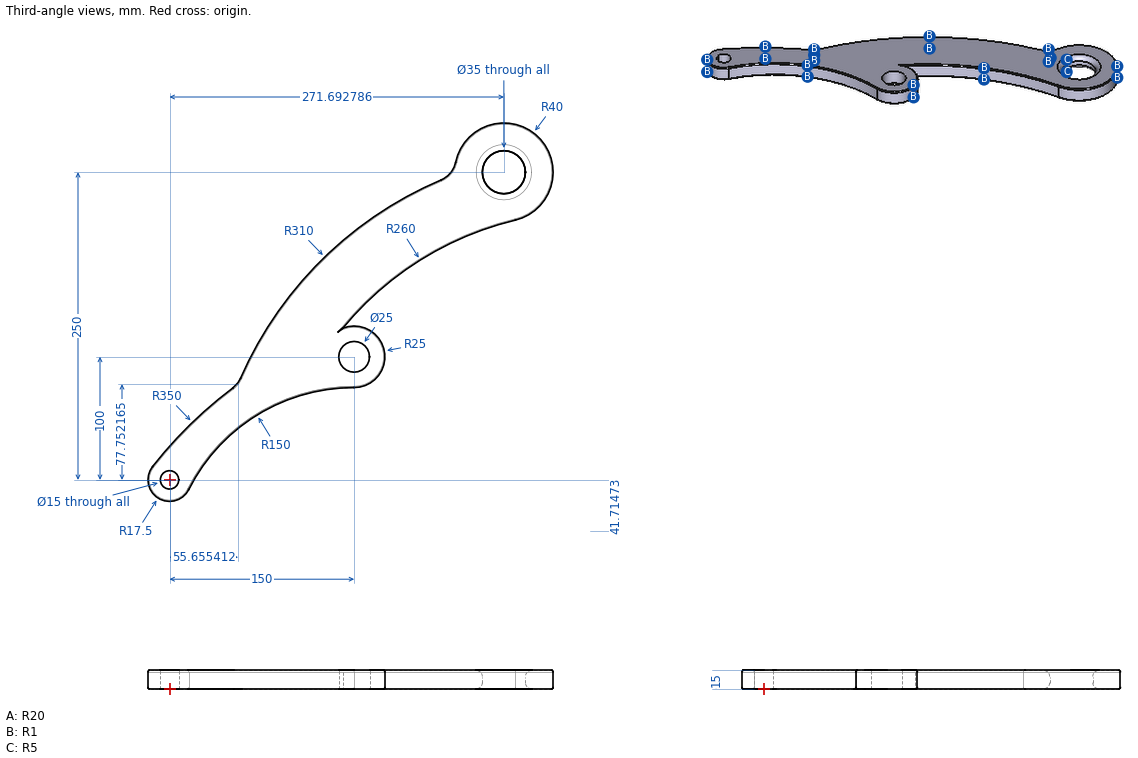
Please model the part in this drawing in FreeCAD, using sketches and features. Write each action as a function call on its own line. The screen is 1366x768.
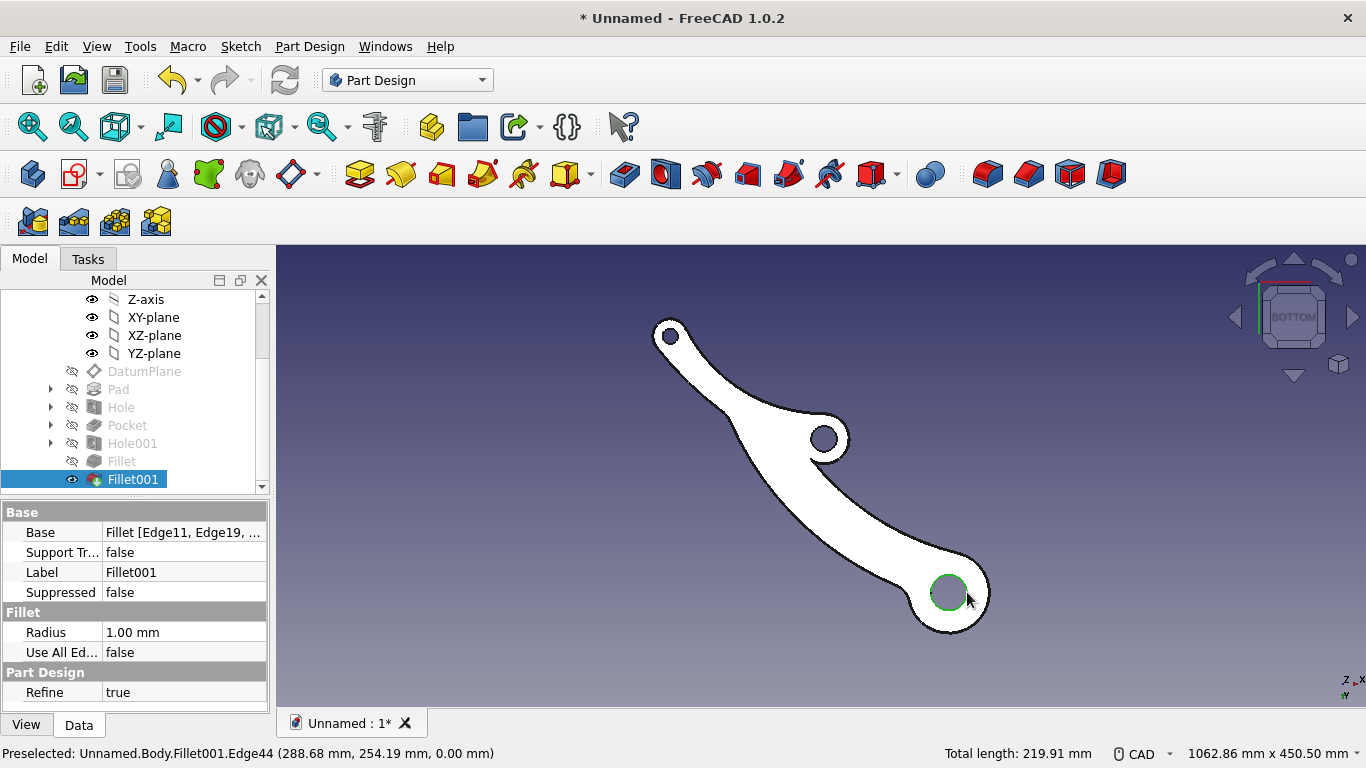
click(988, 174)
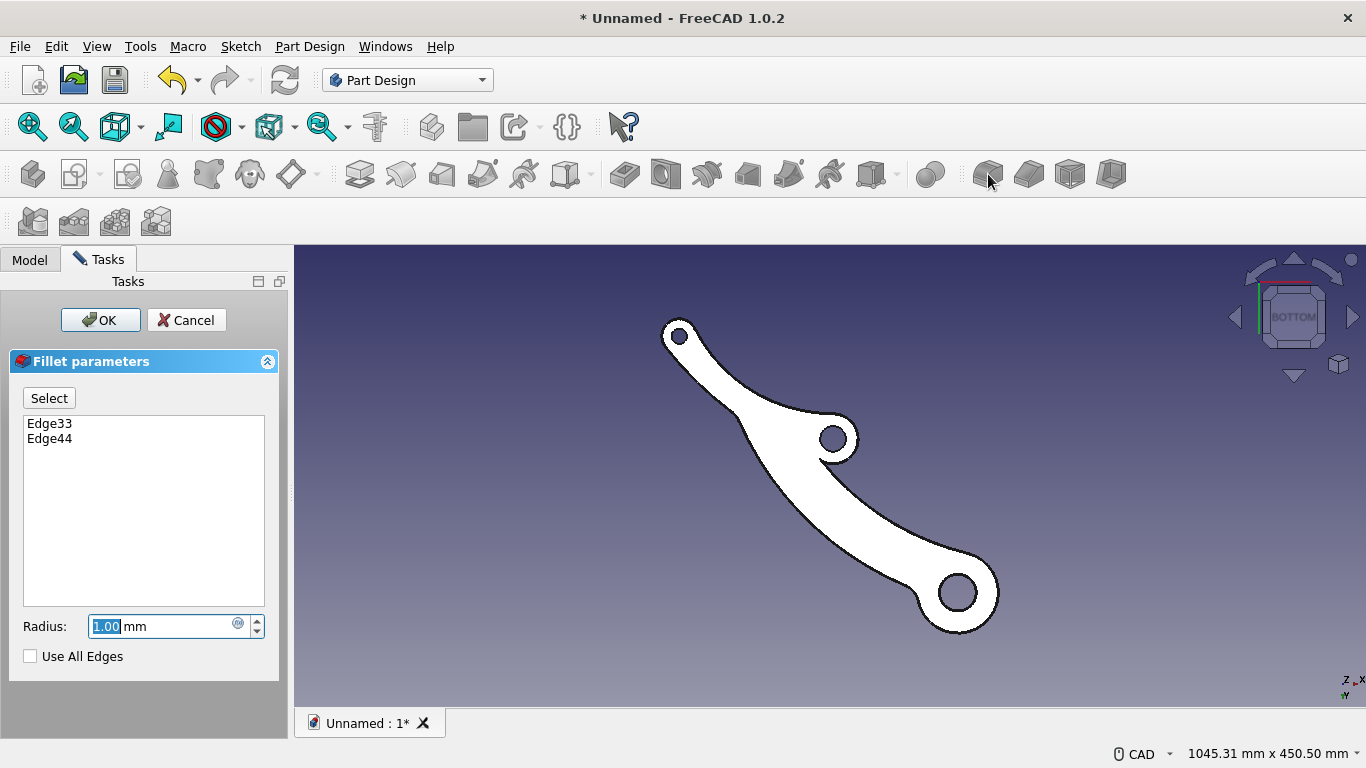
text(5)
key(Tab)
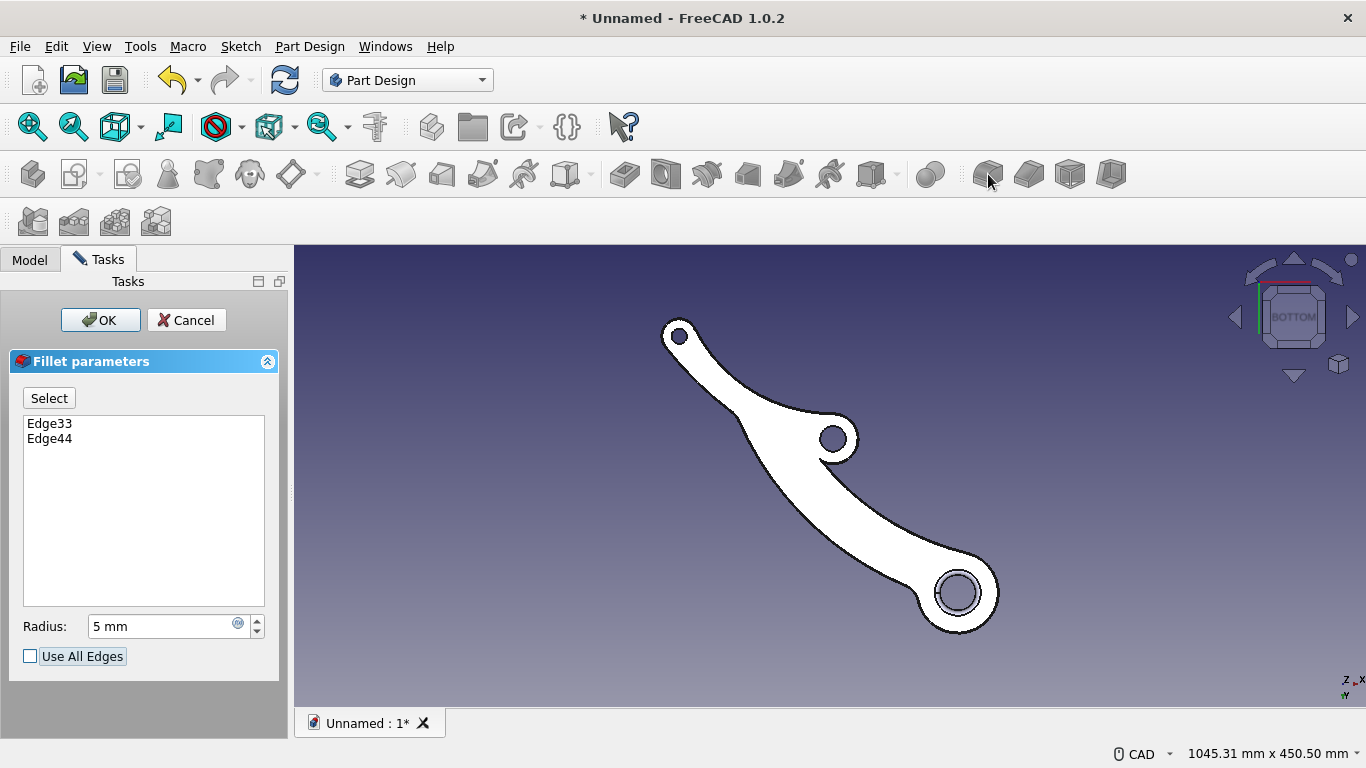
click(101, 320)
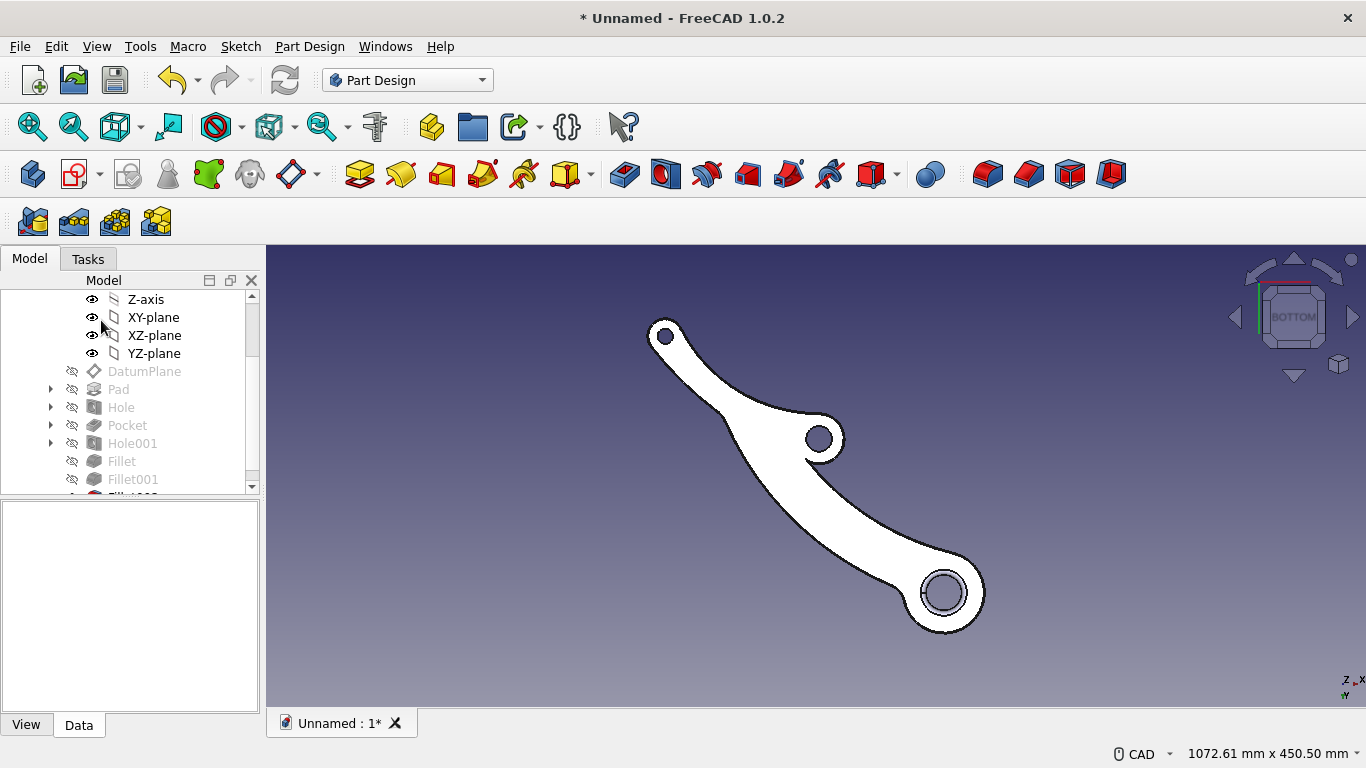
key(0)